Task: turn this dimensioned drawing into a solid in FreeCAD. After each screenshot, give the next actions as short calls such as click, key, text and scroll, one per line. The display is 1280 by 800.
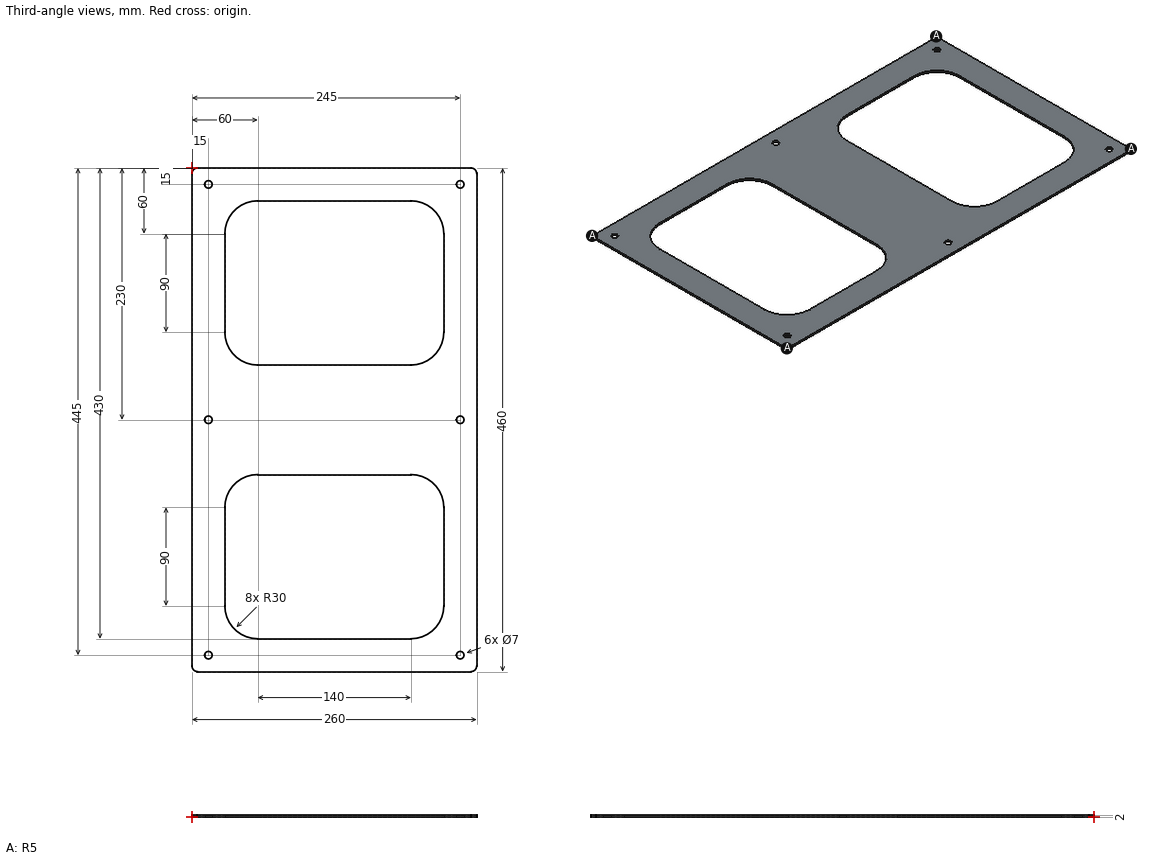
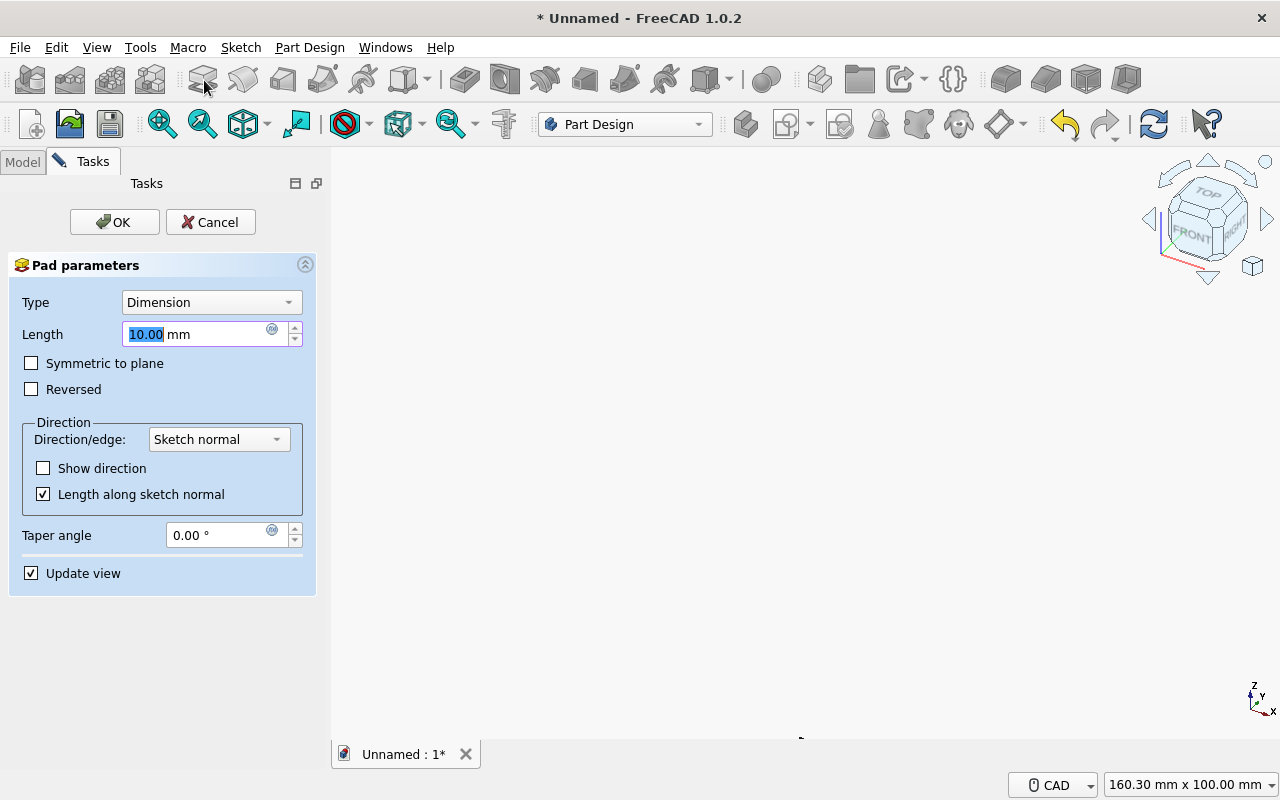
text(2)
key(Tab)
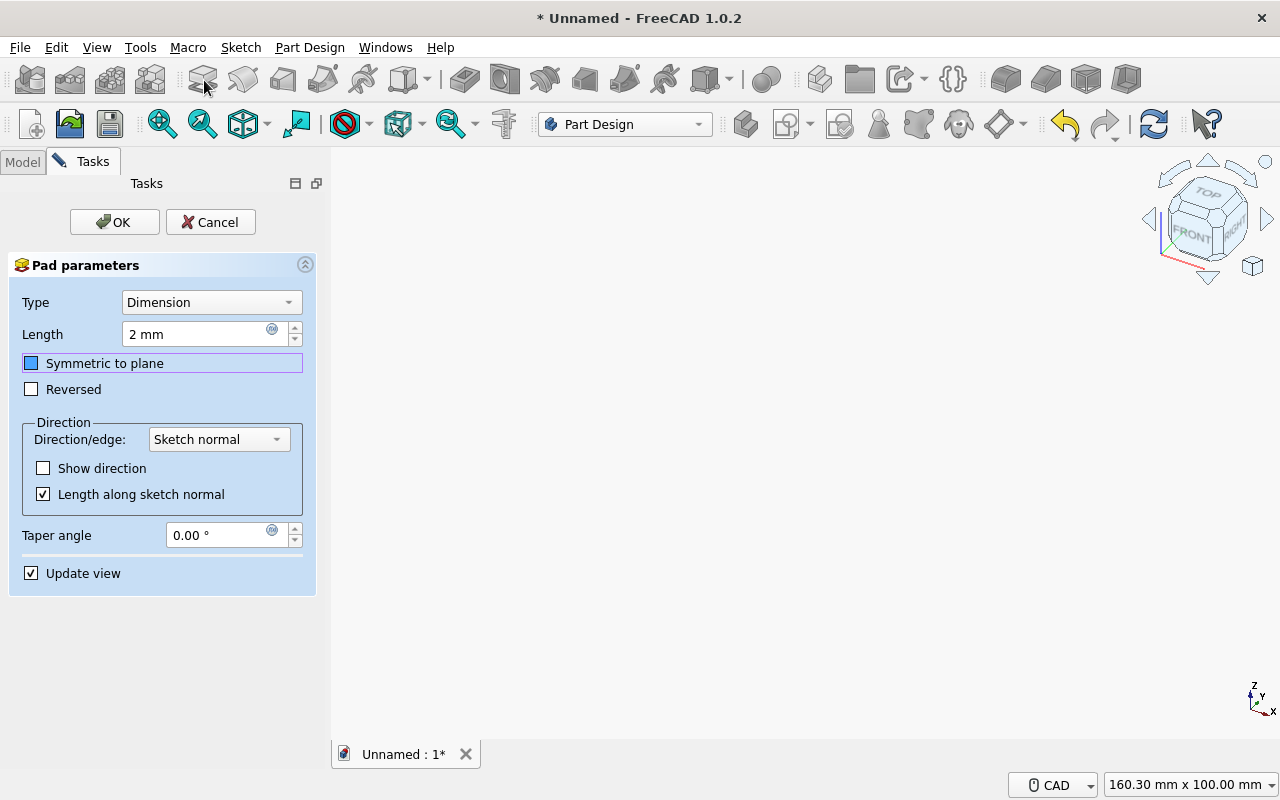
click(115, 222)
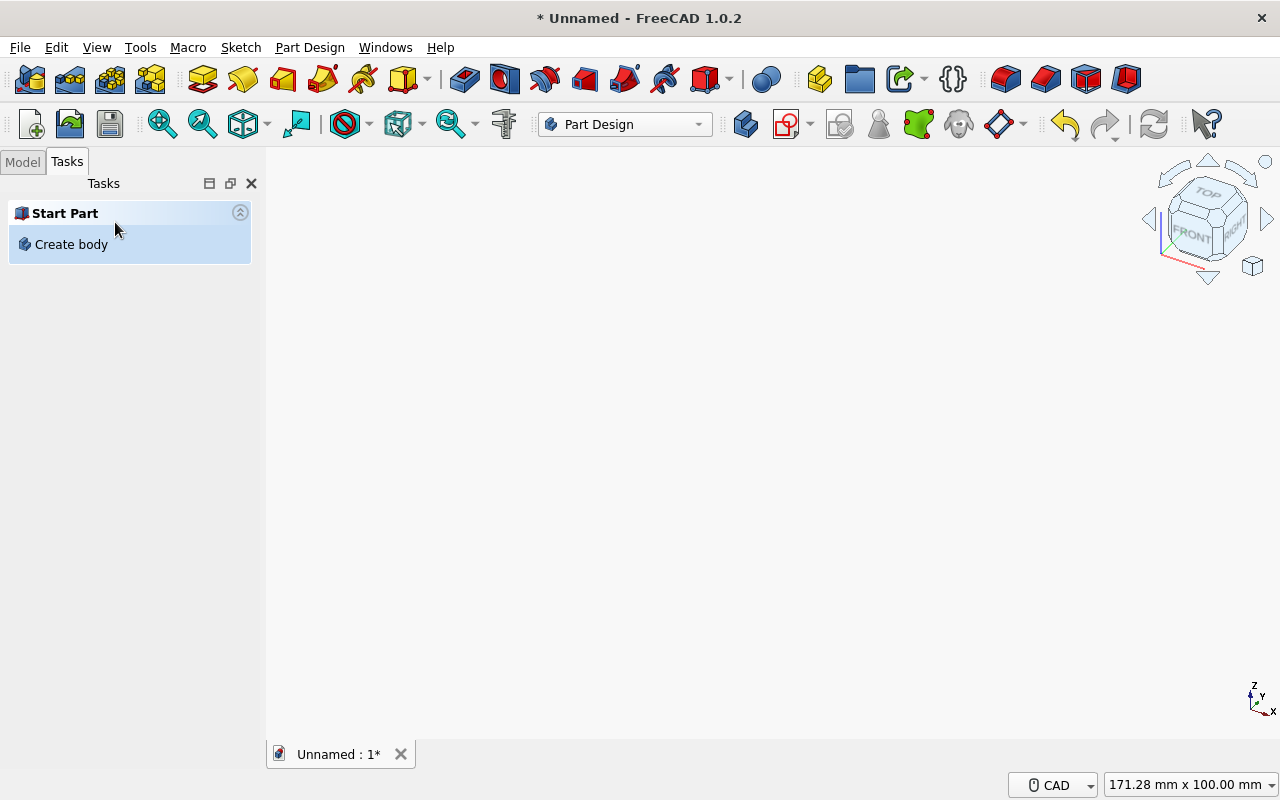
click(164, 124)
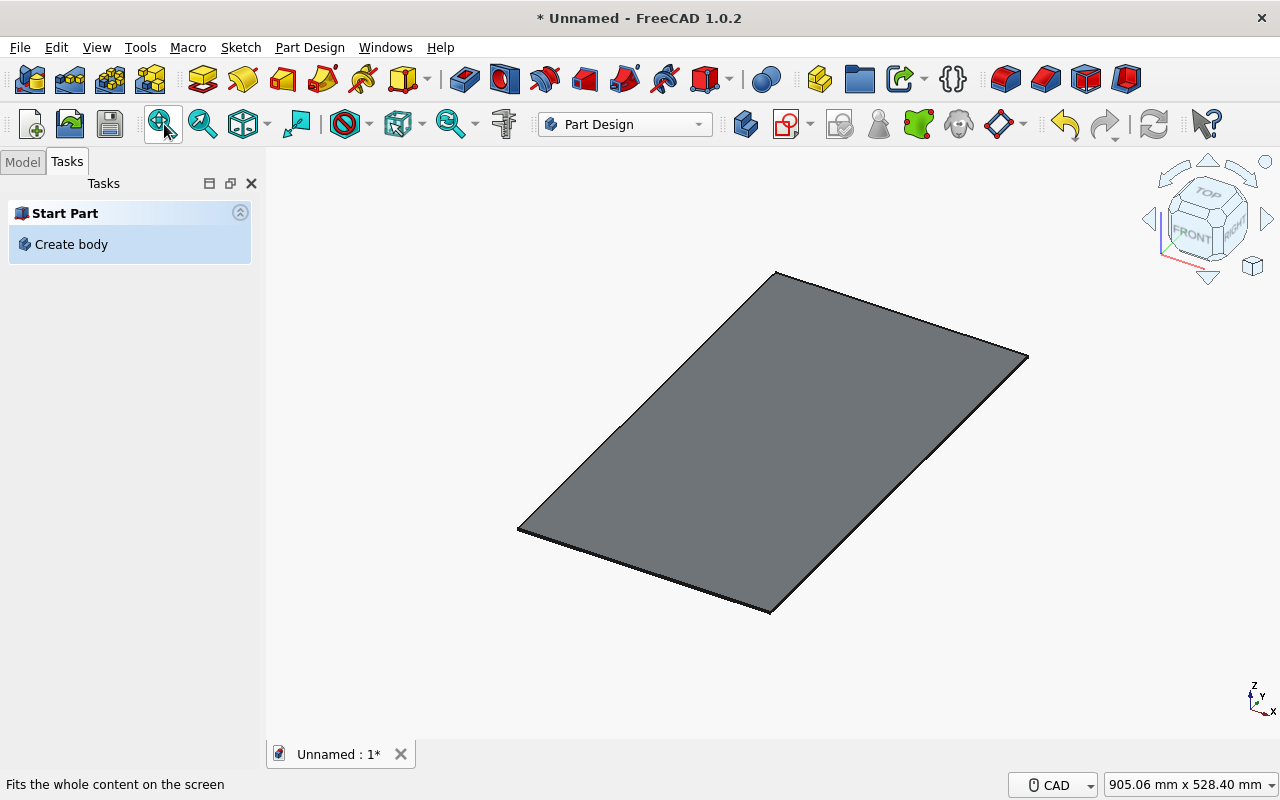
scroll(776, 272, up, 15)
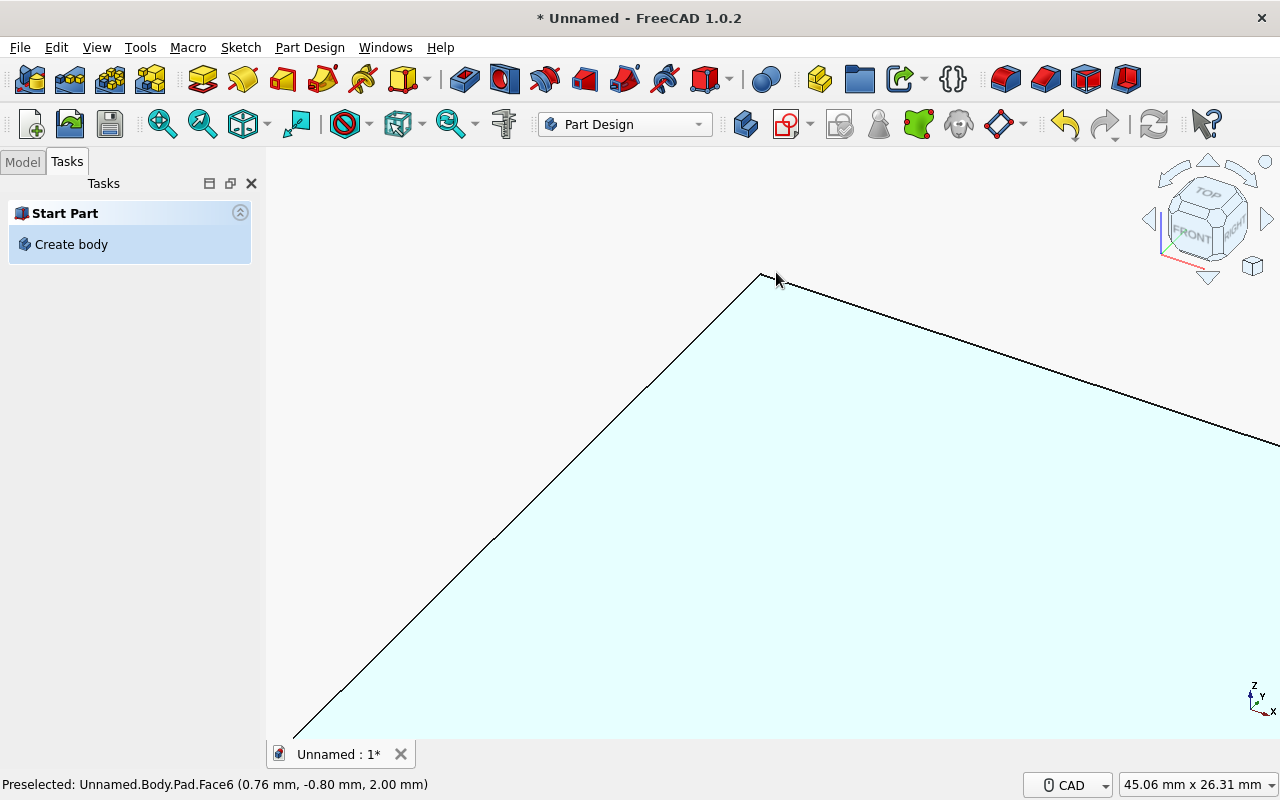
click(164, 124)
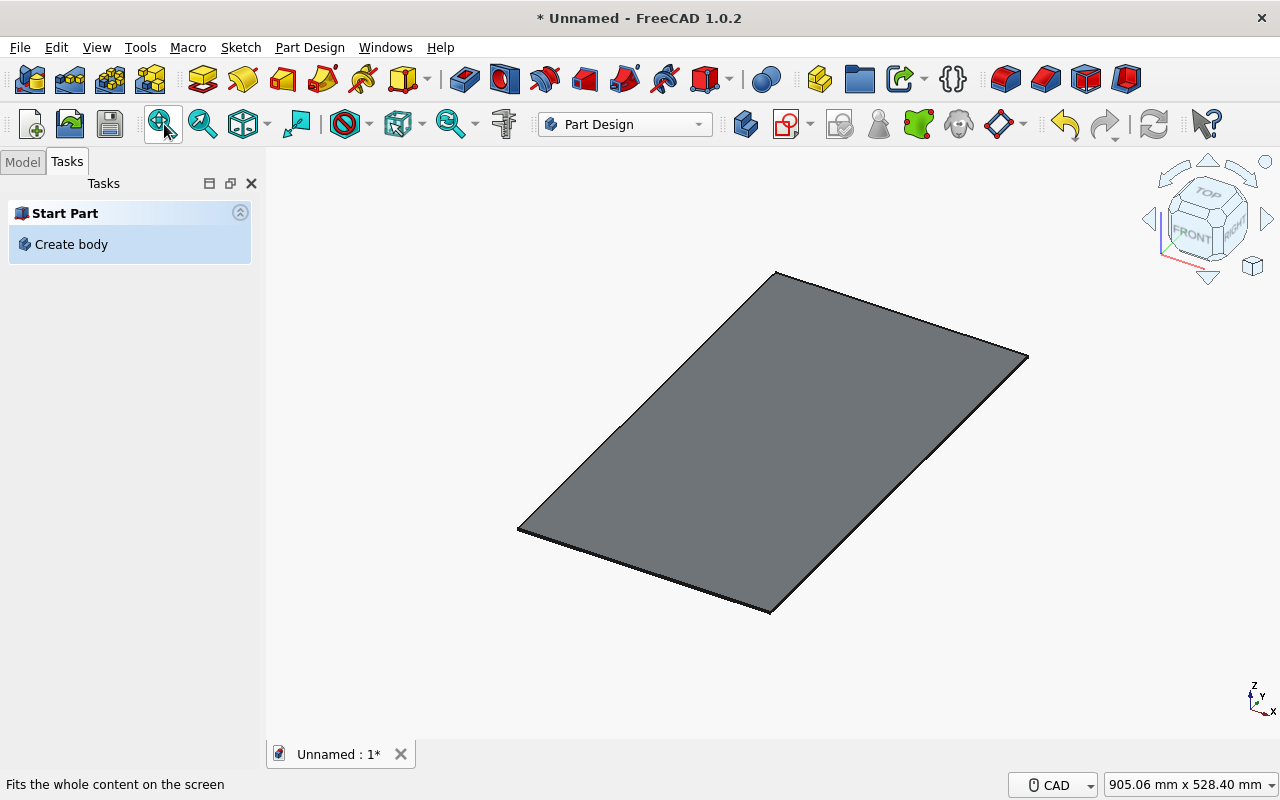
key(0)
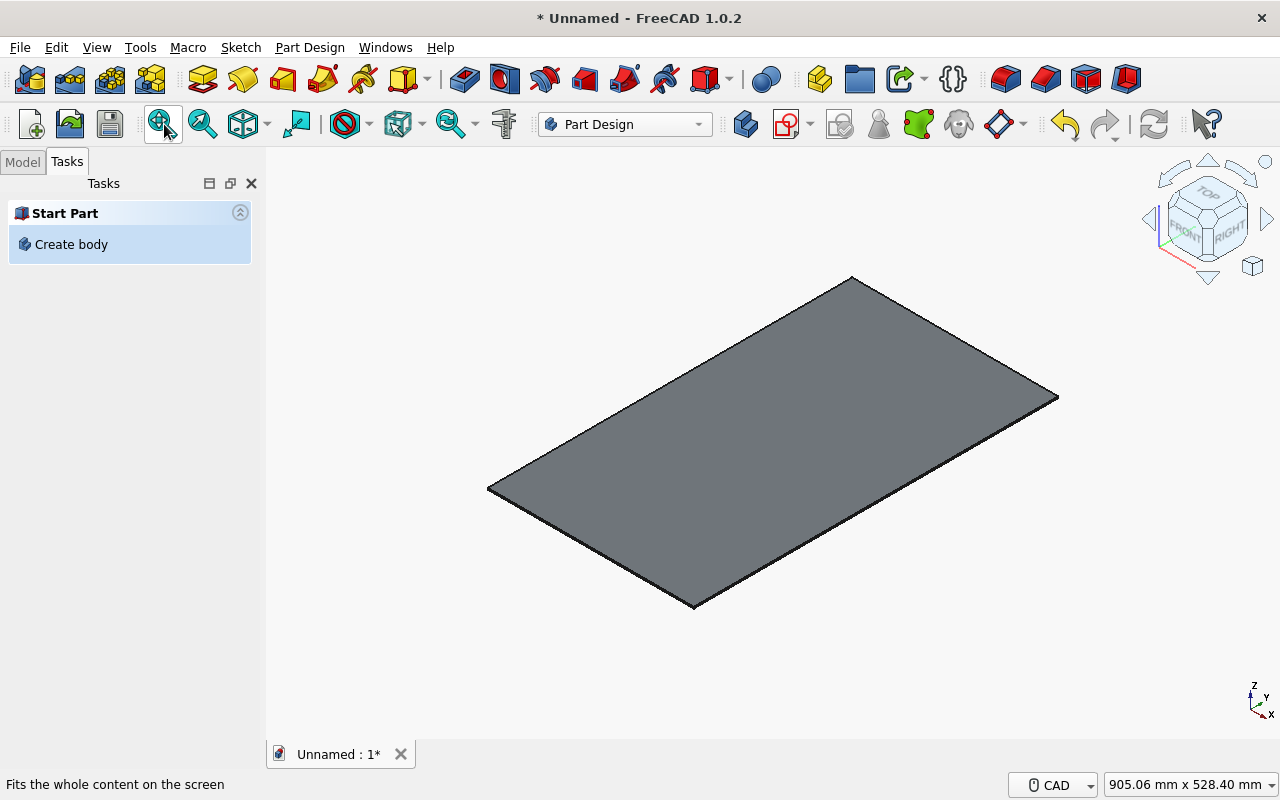
scroll(852, 277, up, 15)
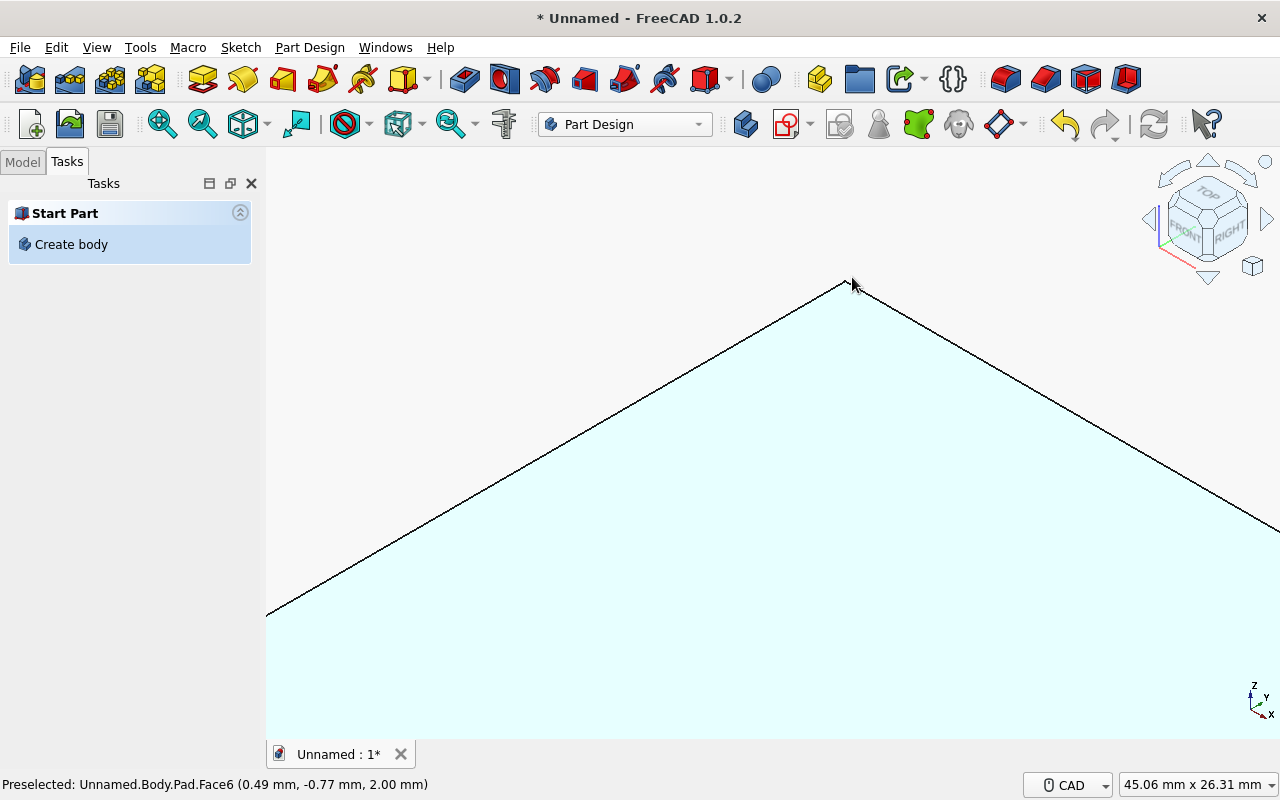
click(164, 124)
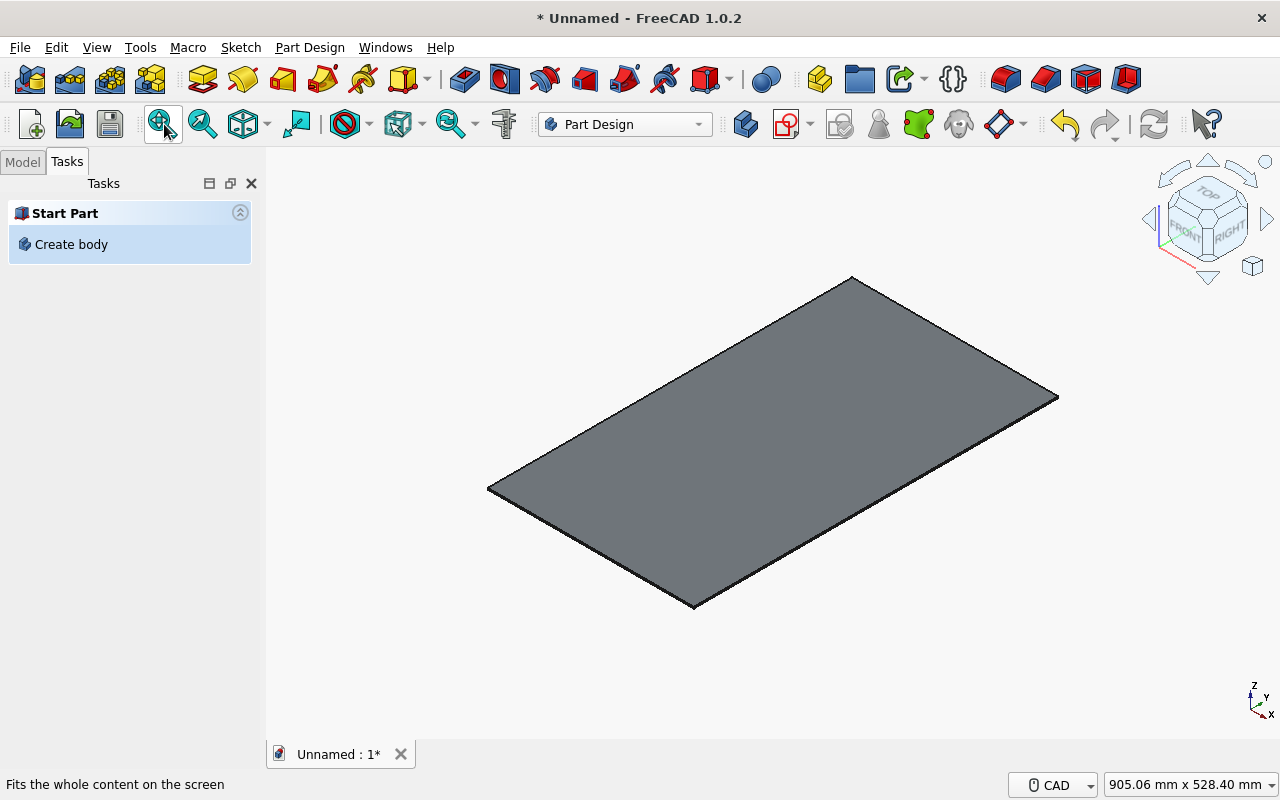
key(2)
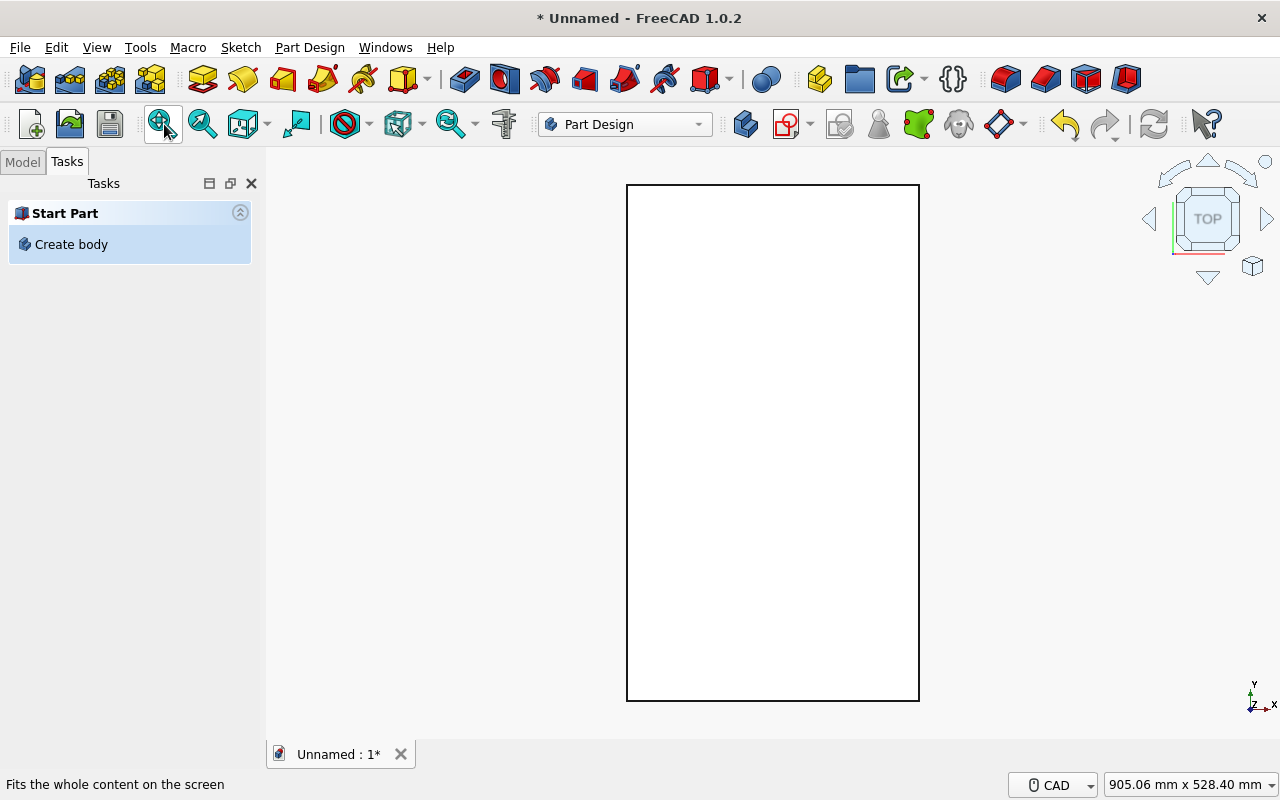
scroll(627, 184, up, 15)